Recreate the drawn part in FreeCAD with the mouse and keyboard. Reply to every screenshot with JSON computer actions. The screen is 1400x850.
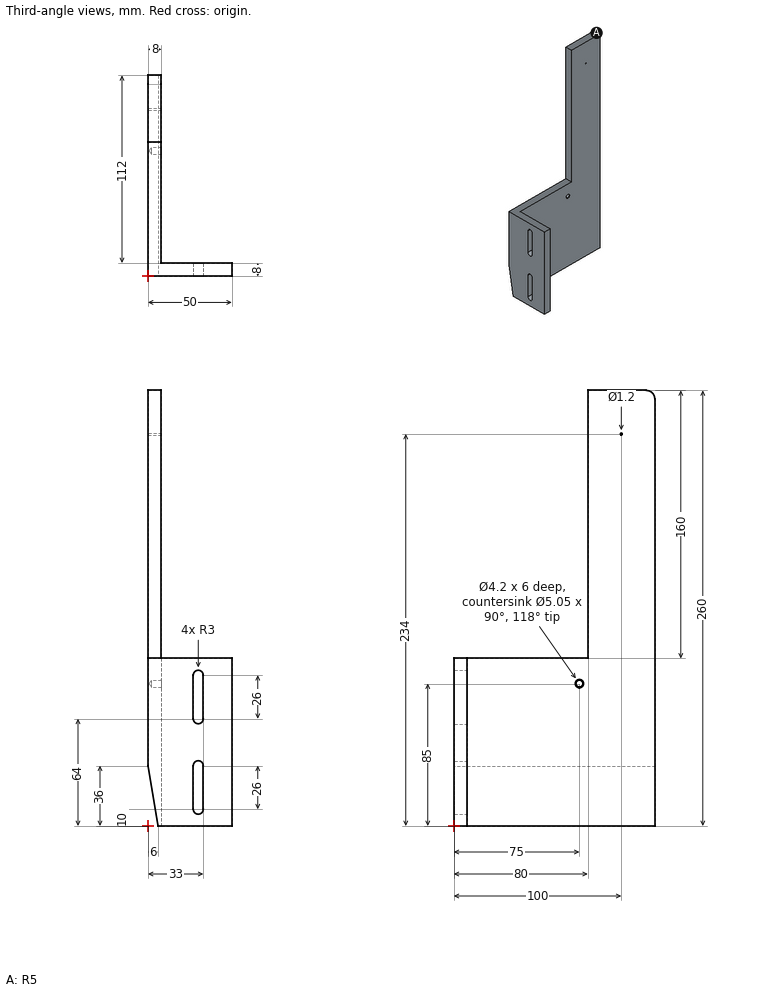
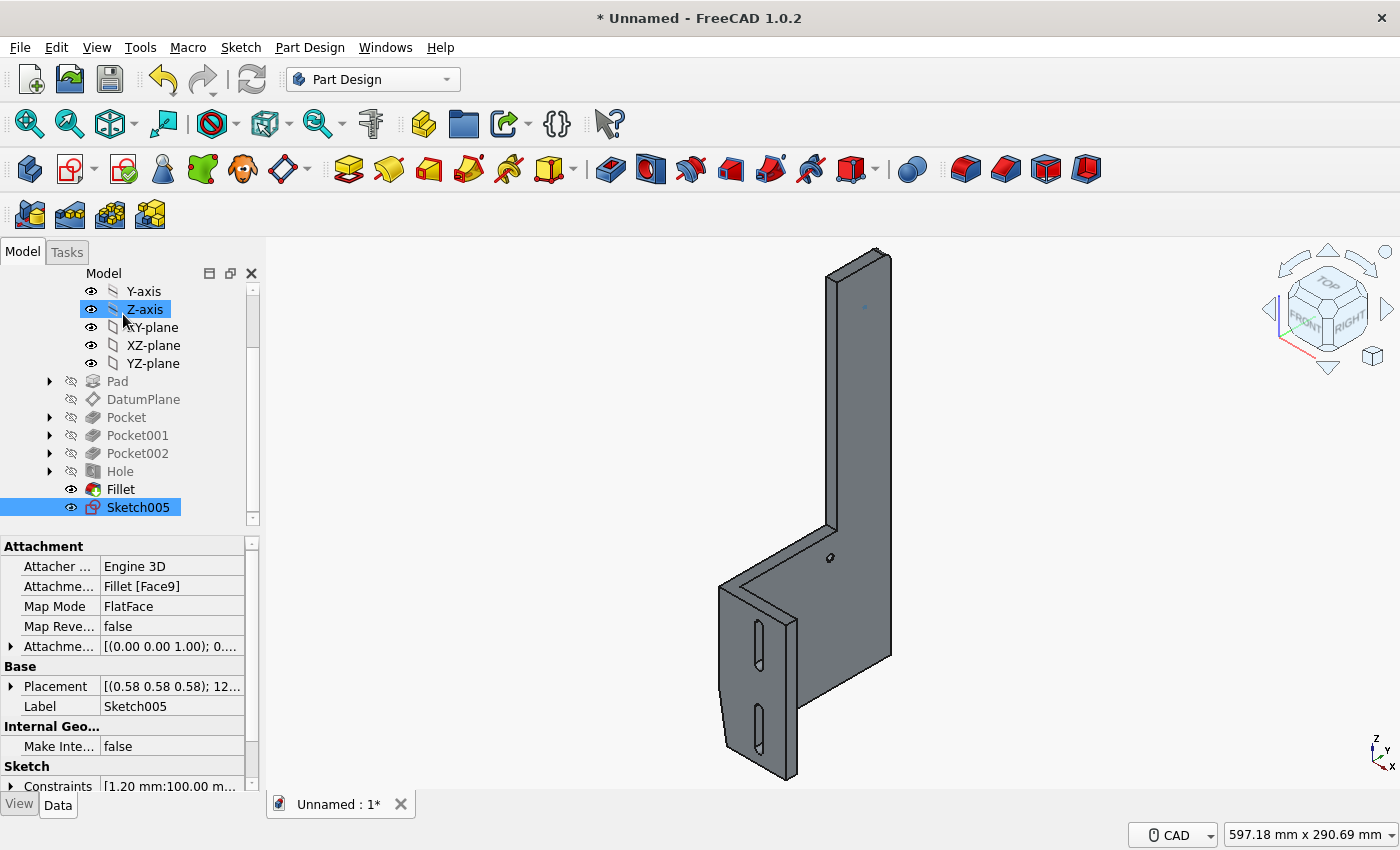
{"action": "left_click", "coordinate": [612, 170]}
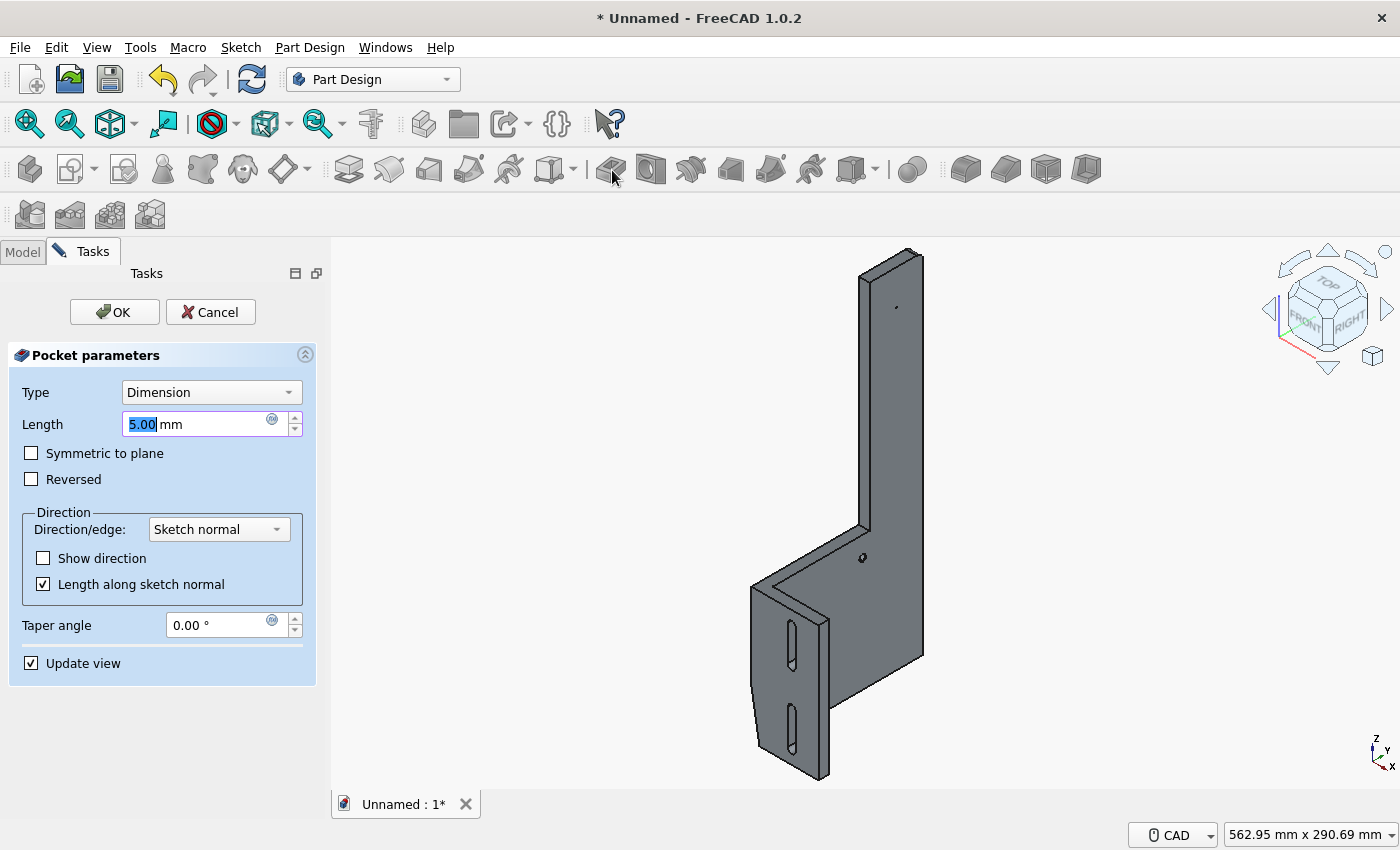
{"action": "left_click", "coordinate": [212, 392]}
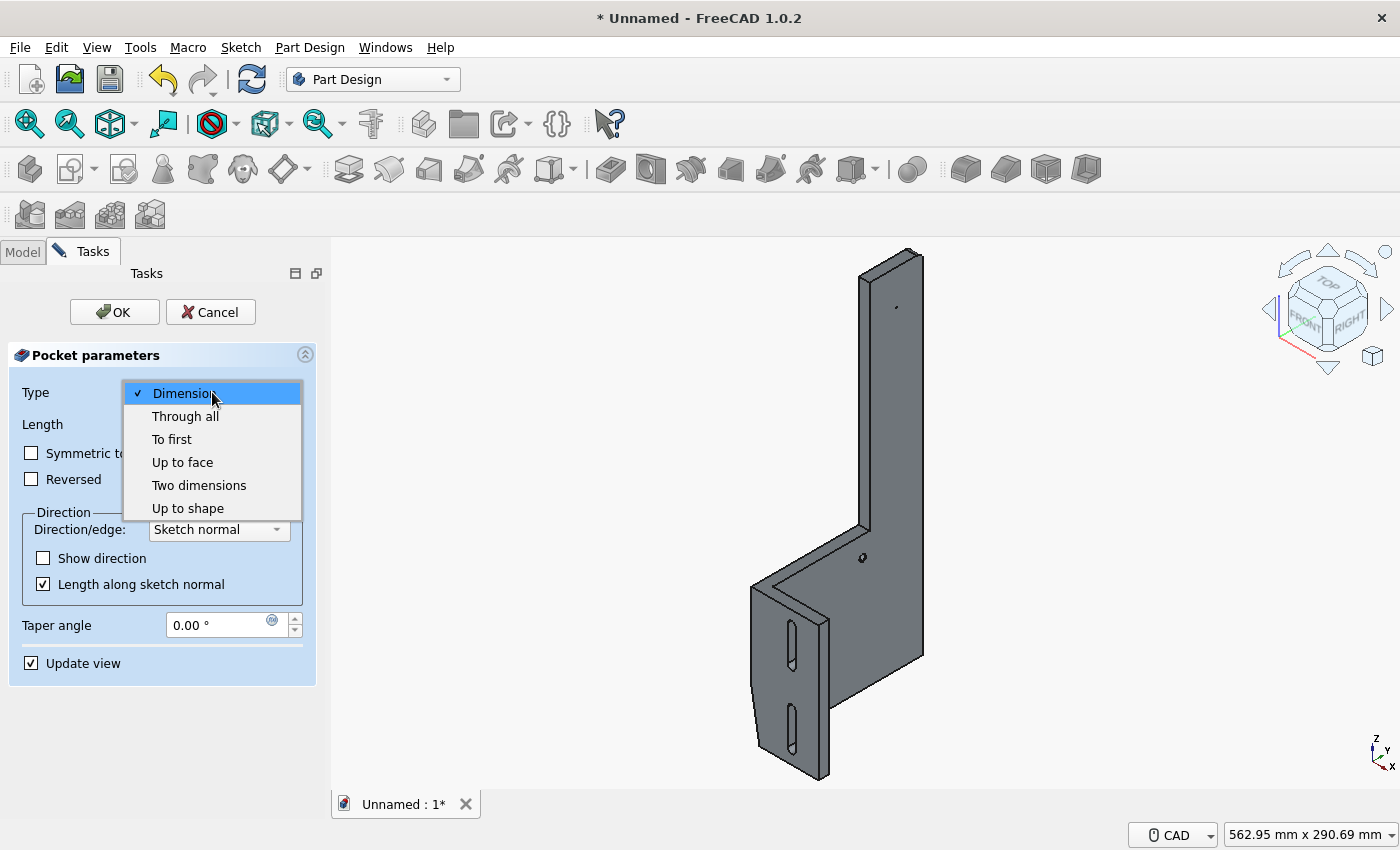
{"action": "left_click", "coordinate": [212, 416]}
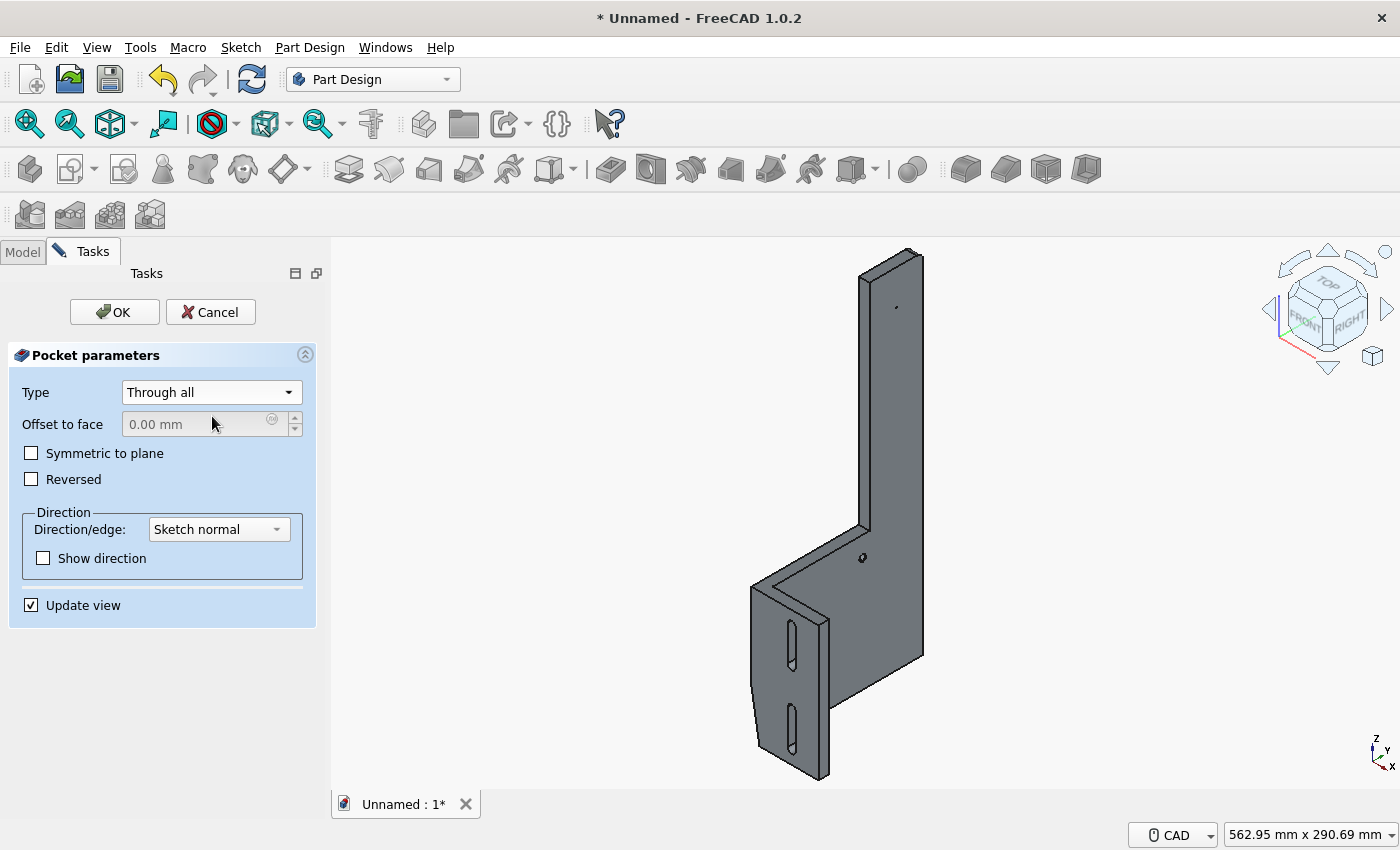
{"action": "left_click", "coordinate": [115, 312]}